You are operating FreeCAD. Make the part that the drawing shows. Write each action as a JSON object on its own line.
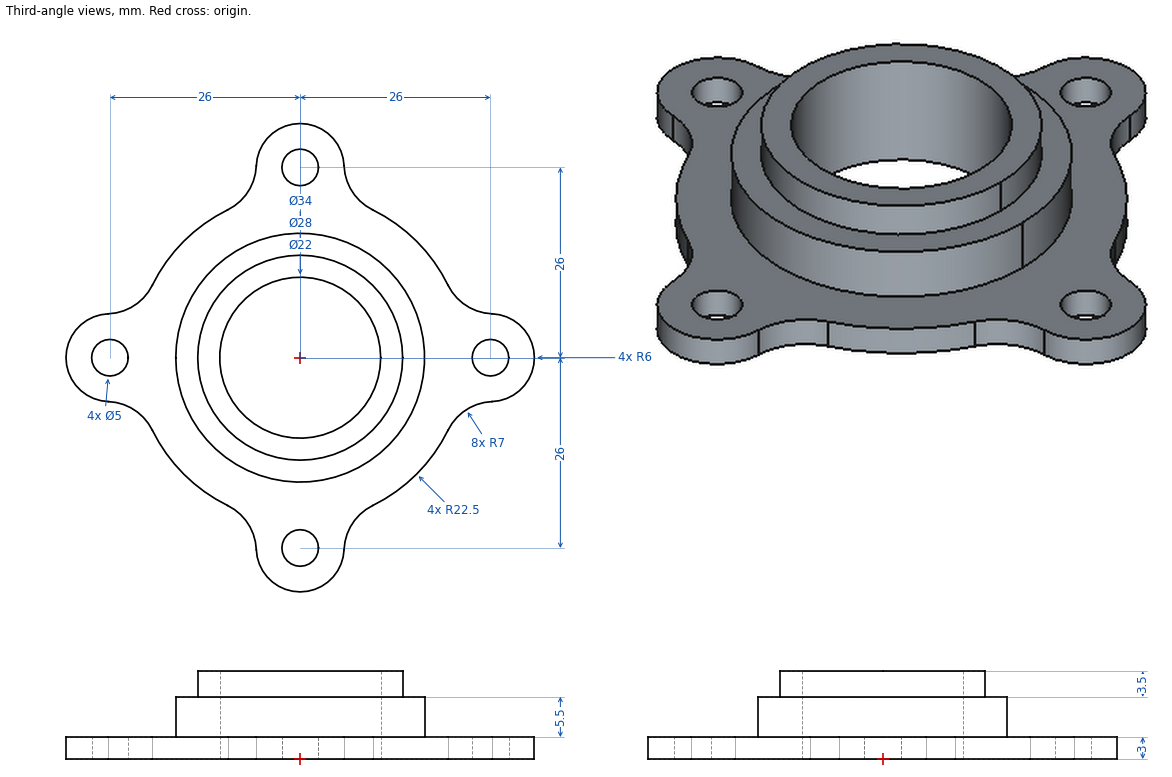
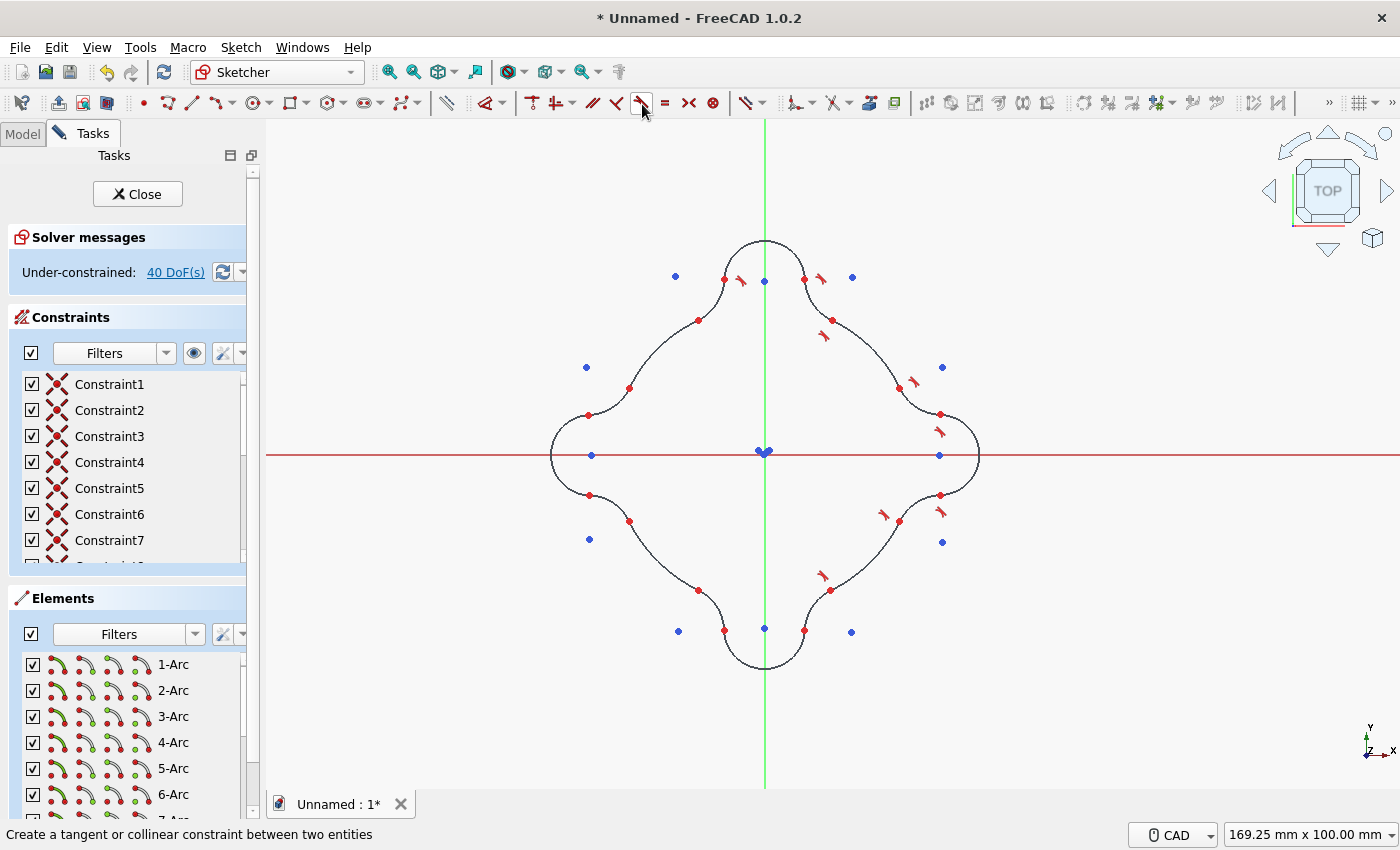
{"action": "left_click", "coordinate": [710, 312]}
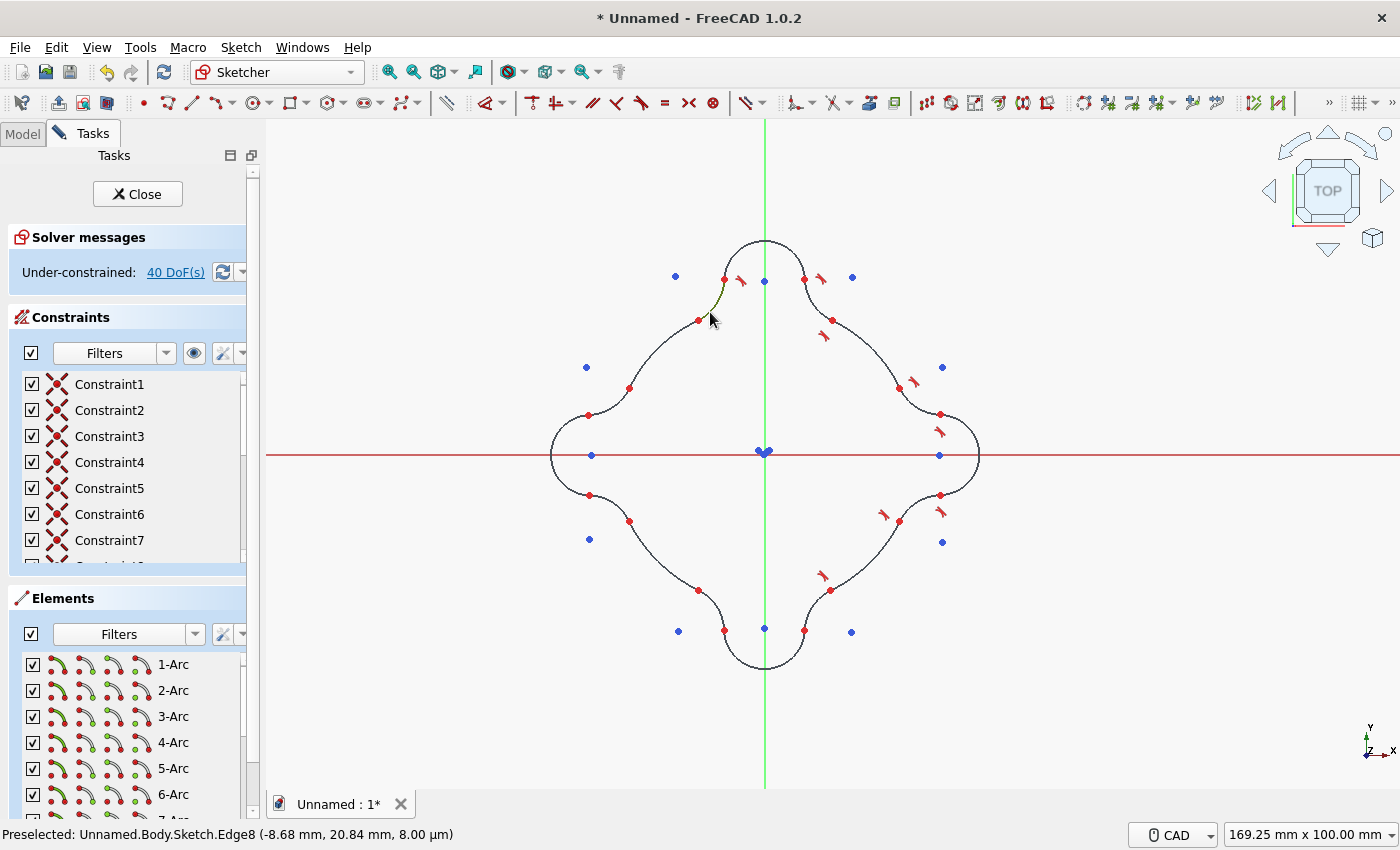
{"action": "left_click", "coordinate": [673, 336]}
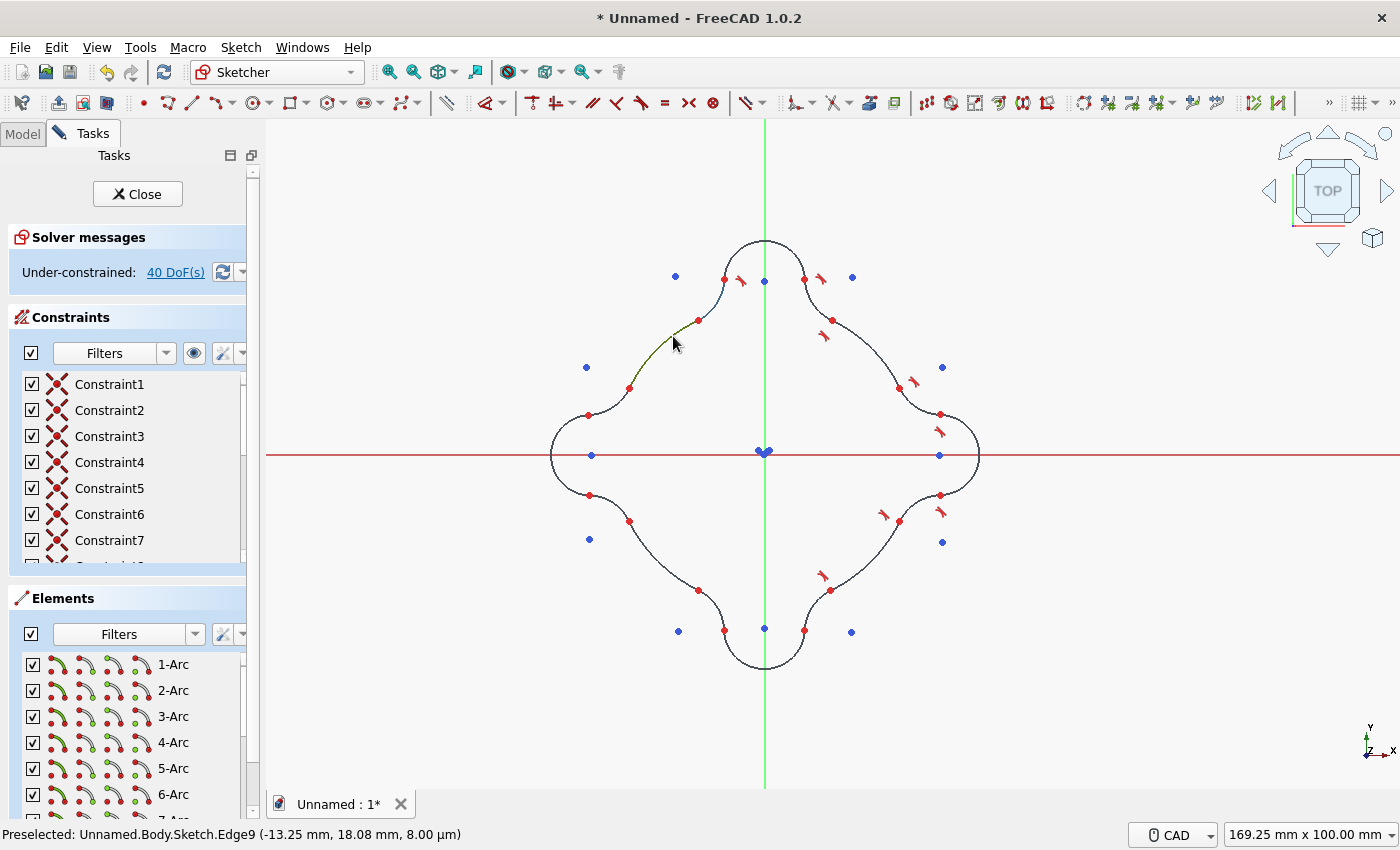
{"action": "left_click", "coordinate": [642, 104]}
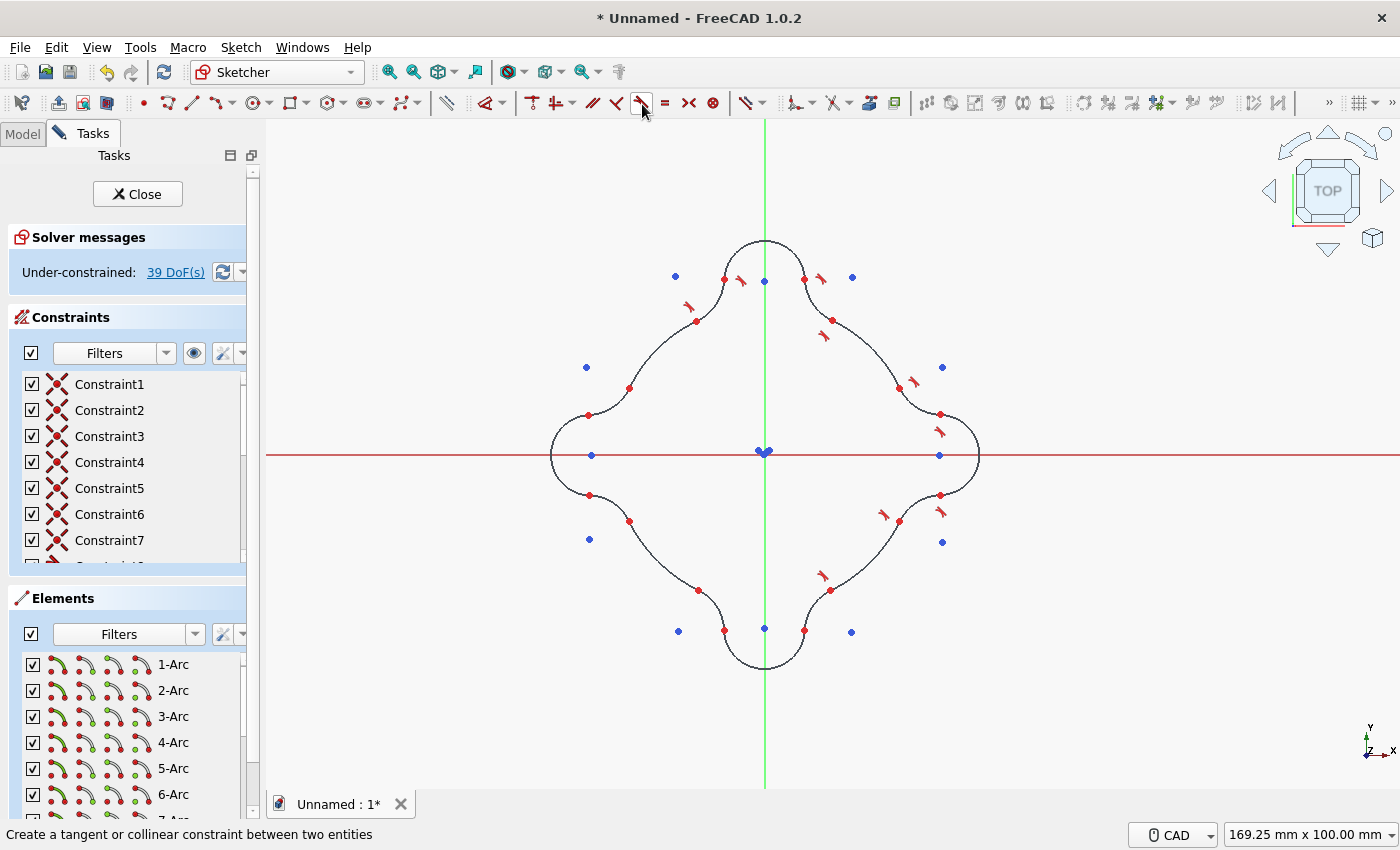
{"action": "left_click", "coordinate": [672, 336]}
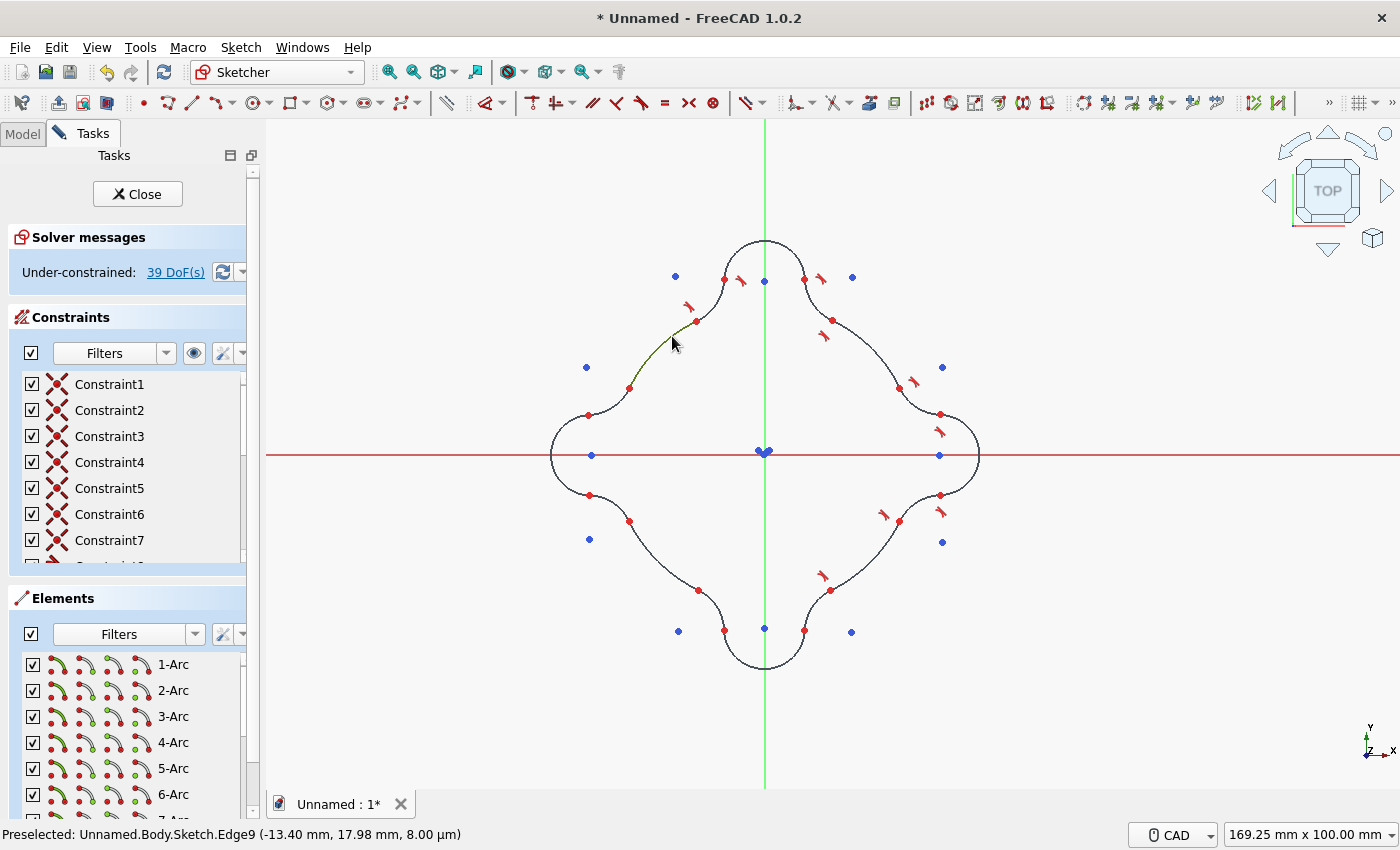
{"action": "left_click", "coordinate": [604, 412]}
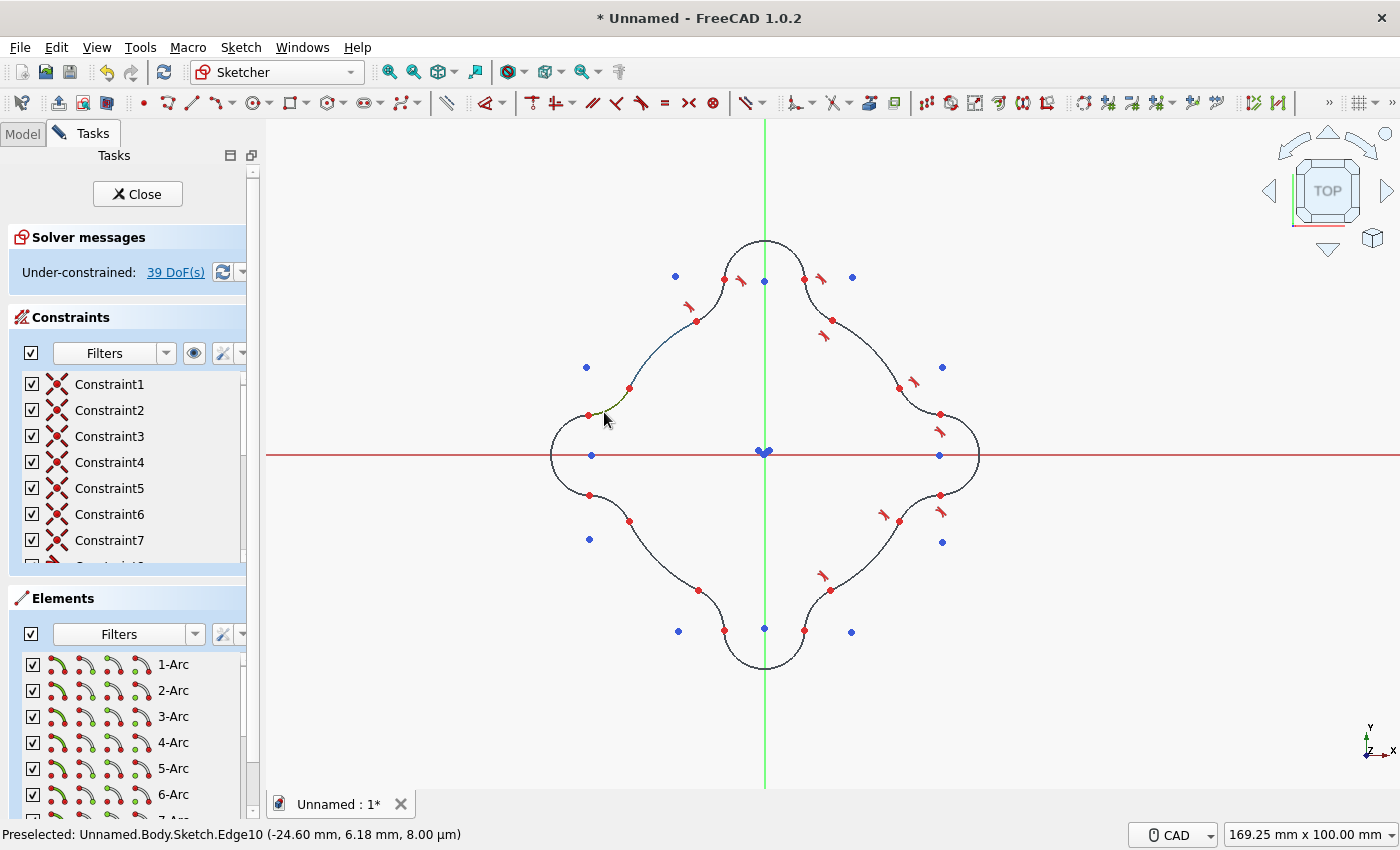
{"action": "left_click", "coordinate": [642, 104]}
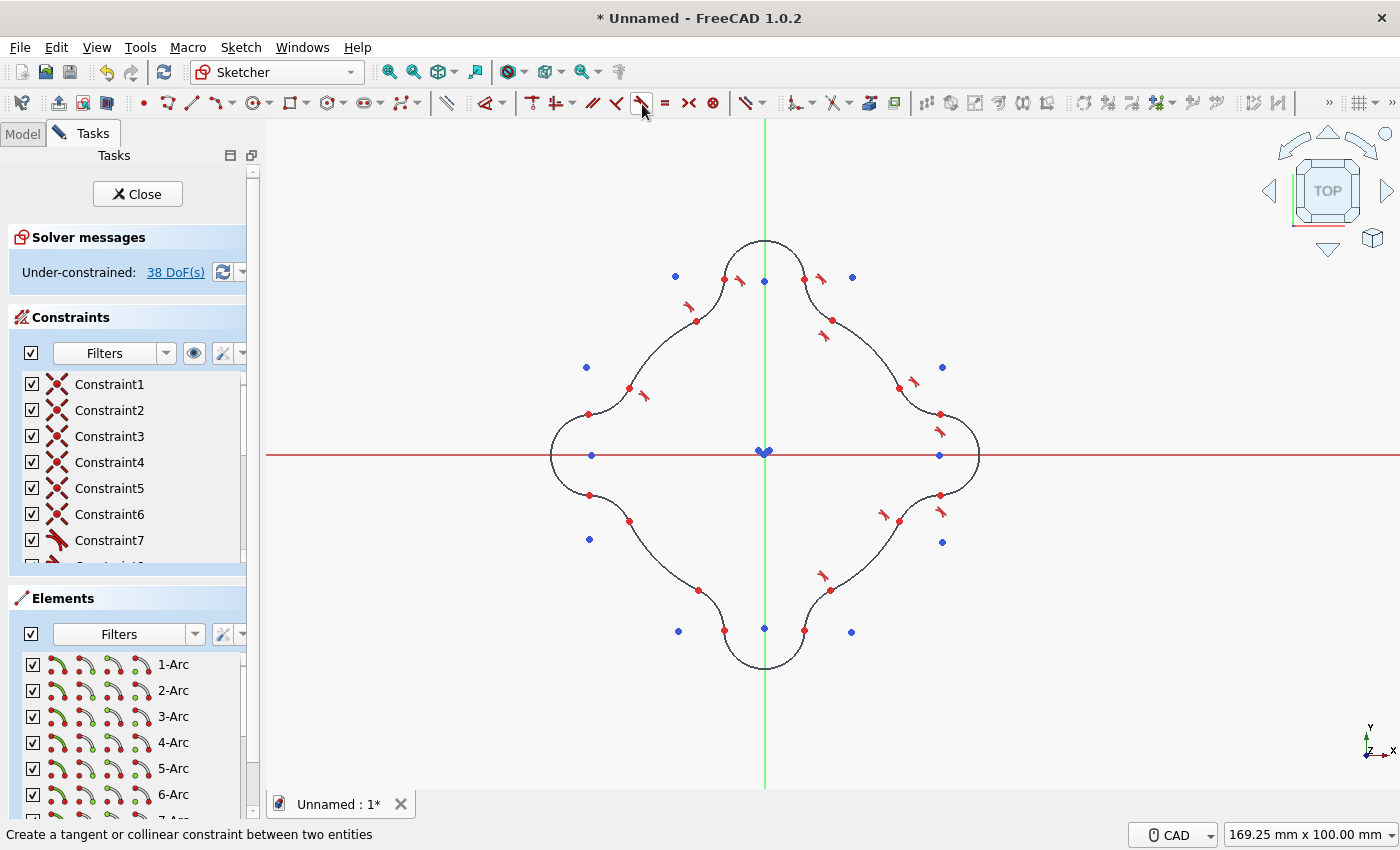
{"action": "left_click", "coordinate": [604, 412]}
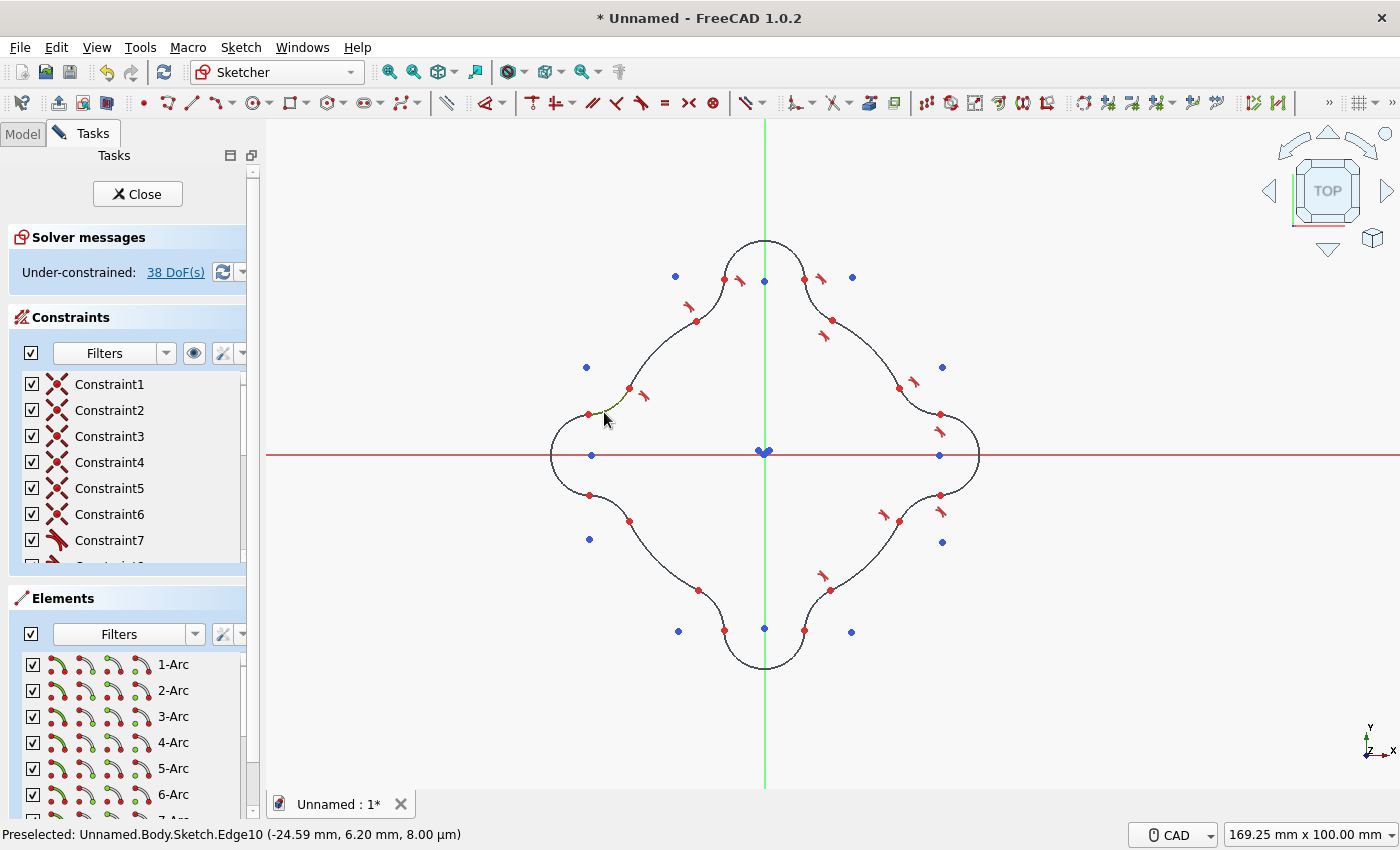
{"action": "left_click", "coordinate": [558, 432]}